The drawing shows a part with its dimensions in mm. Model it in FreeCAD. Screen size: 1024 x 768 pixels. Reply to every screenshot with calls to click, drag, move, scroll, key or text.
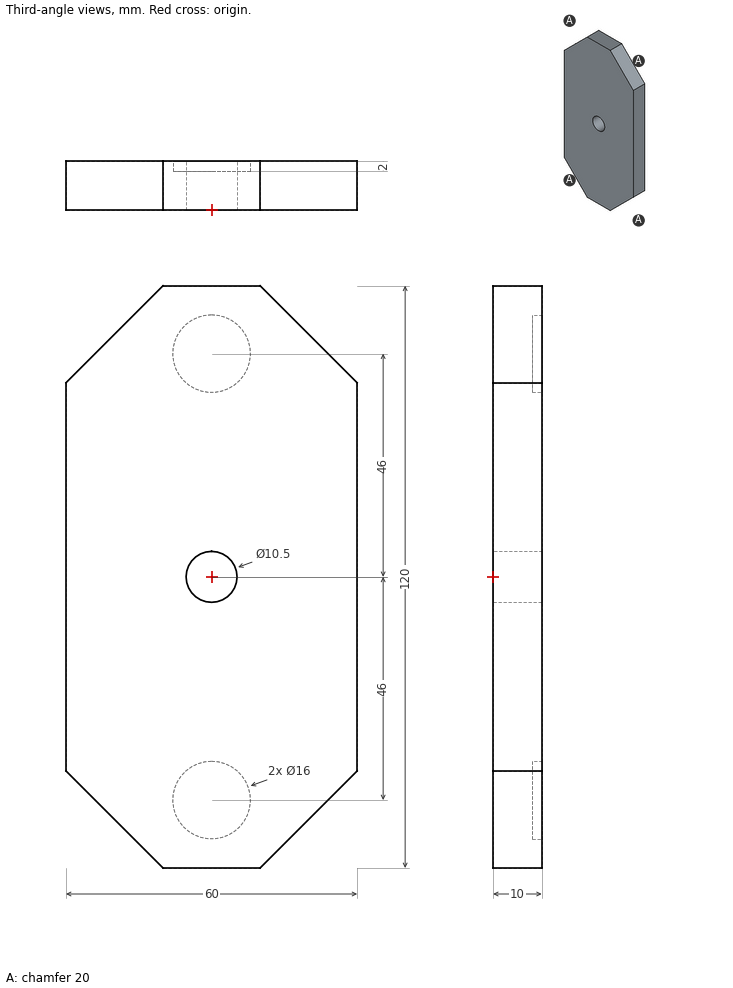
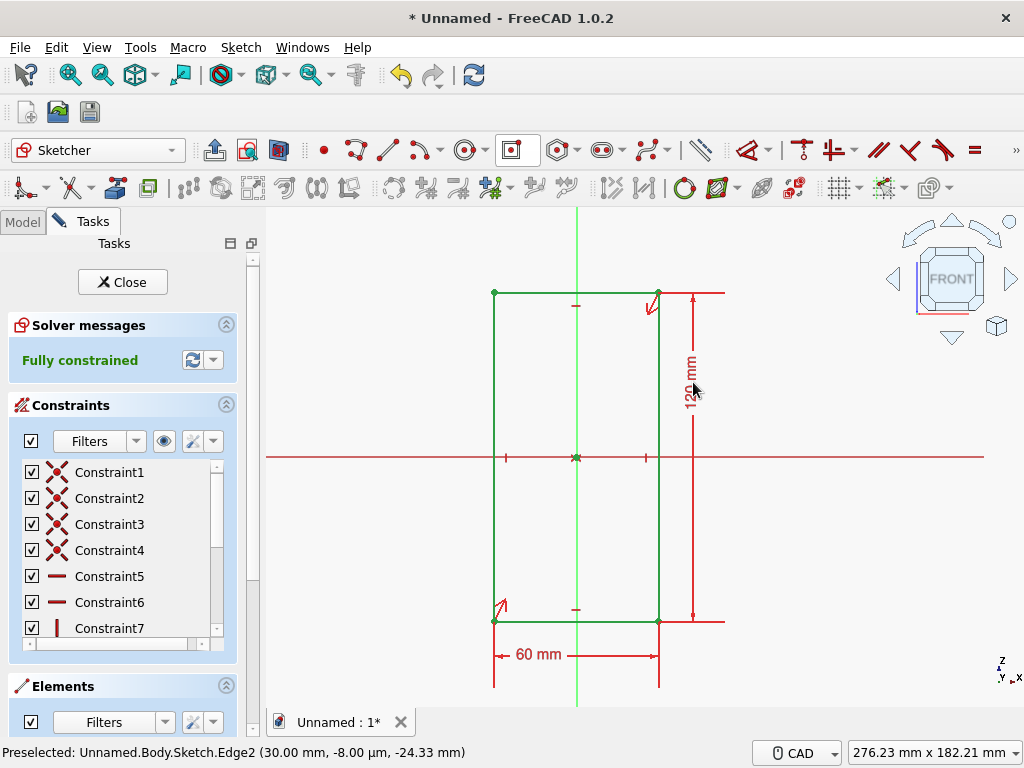
click(123, 282)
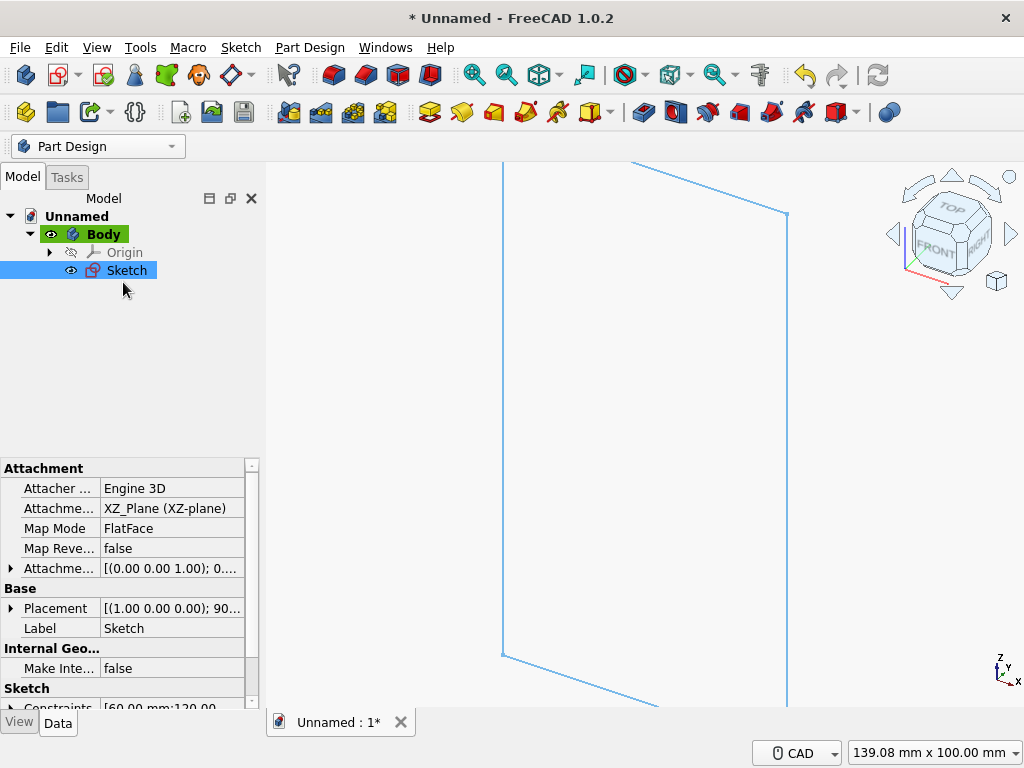
click(430, 112)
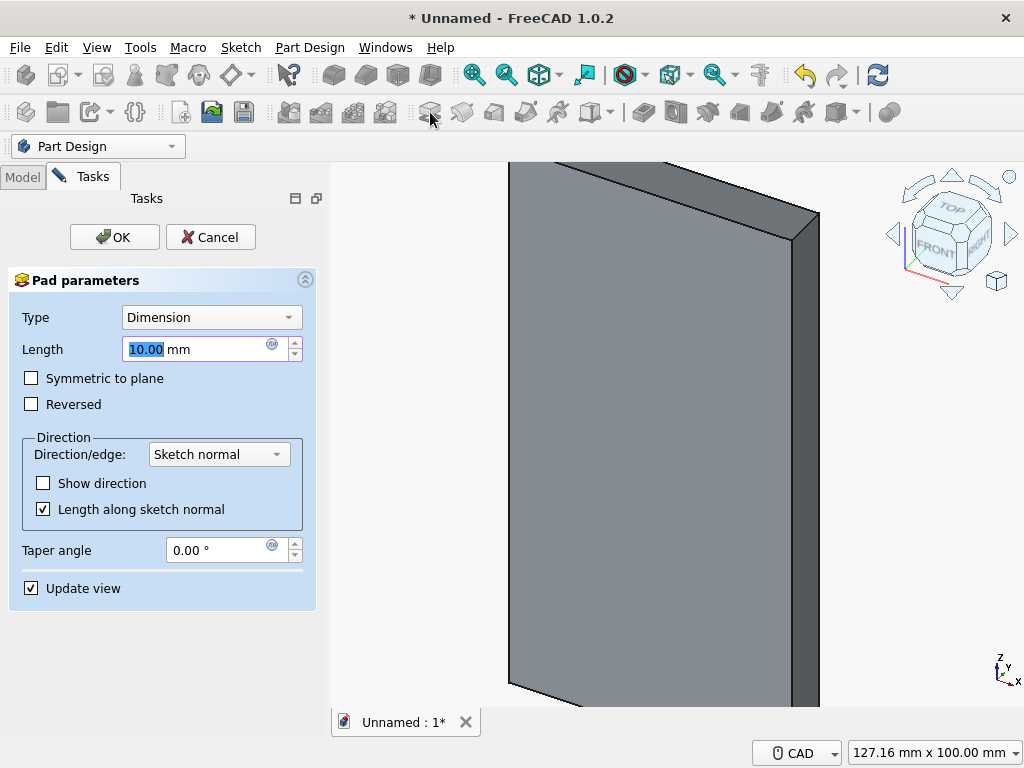
text(10)
key(Tab)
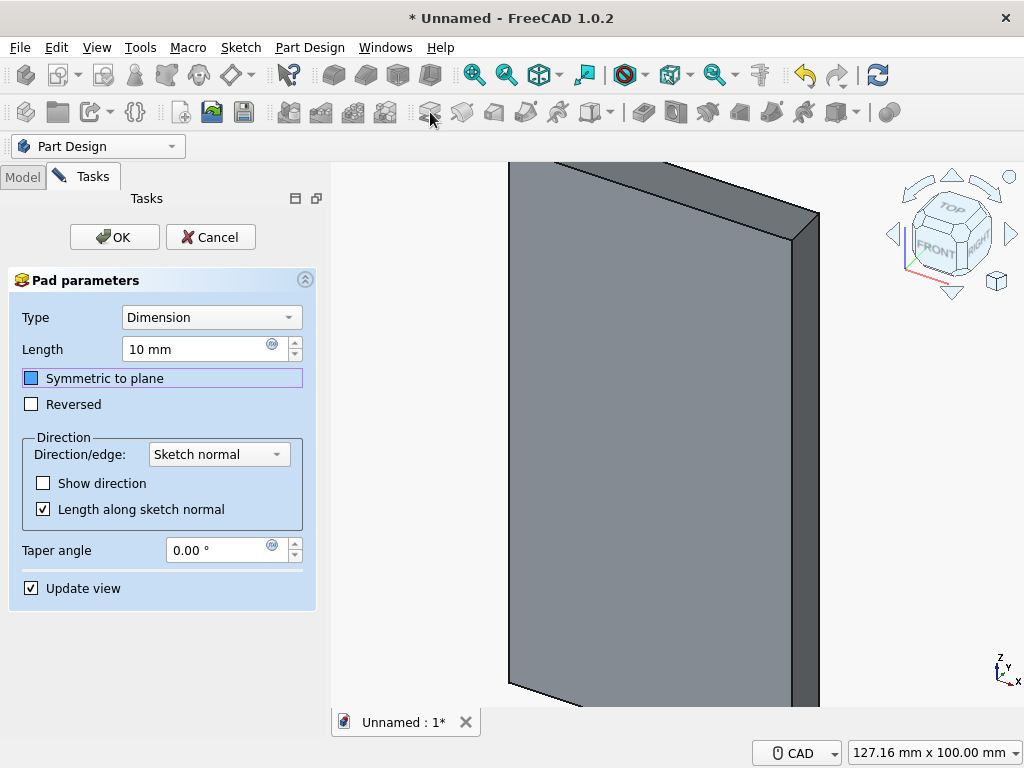
click(30, 404)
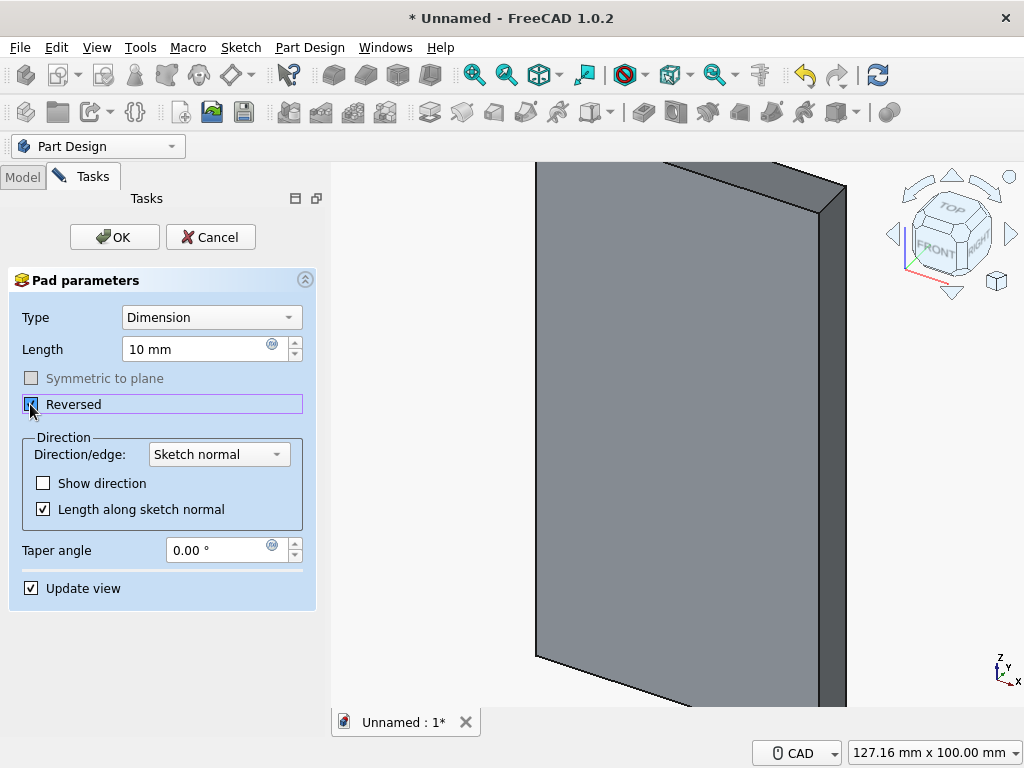
click(115, 237)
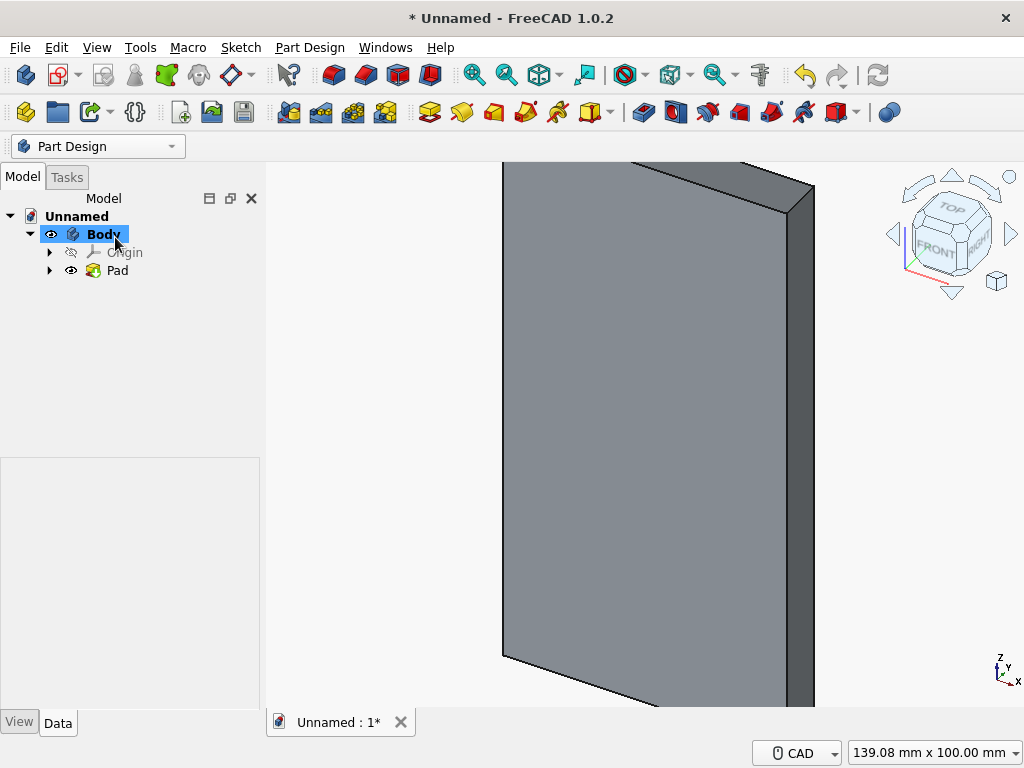
click(476, 76)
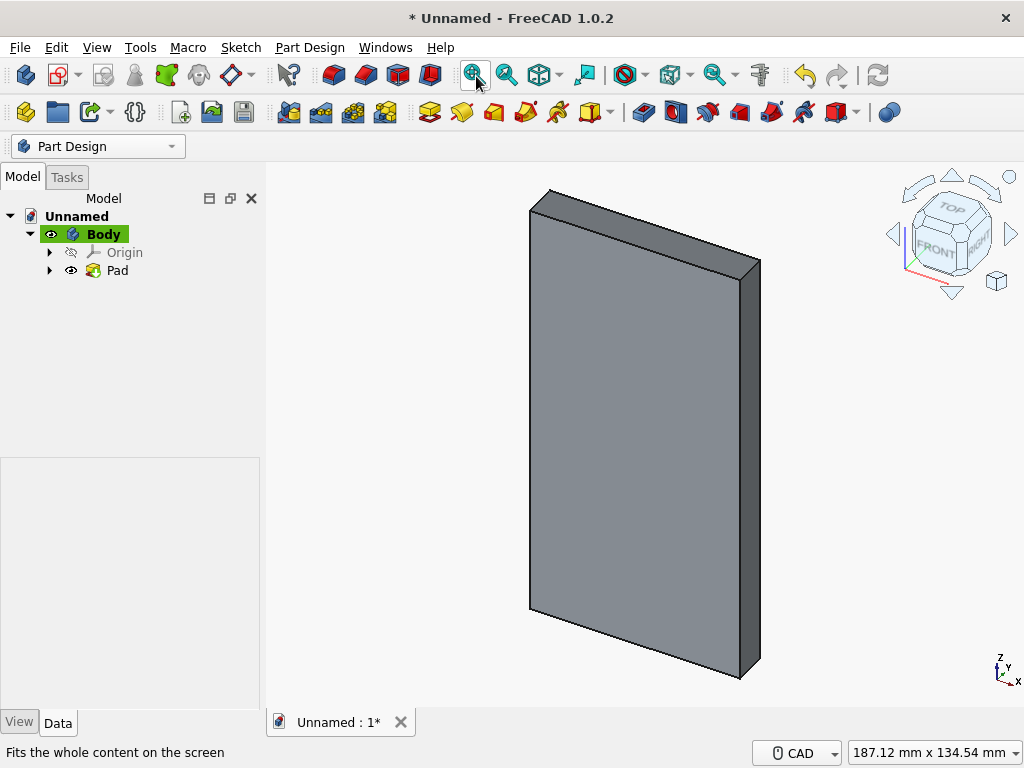
key(4)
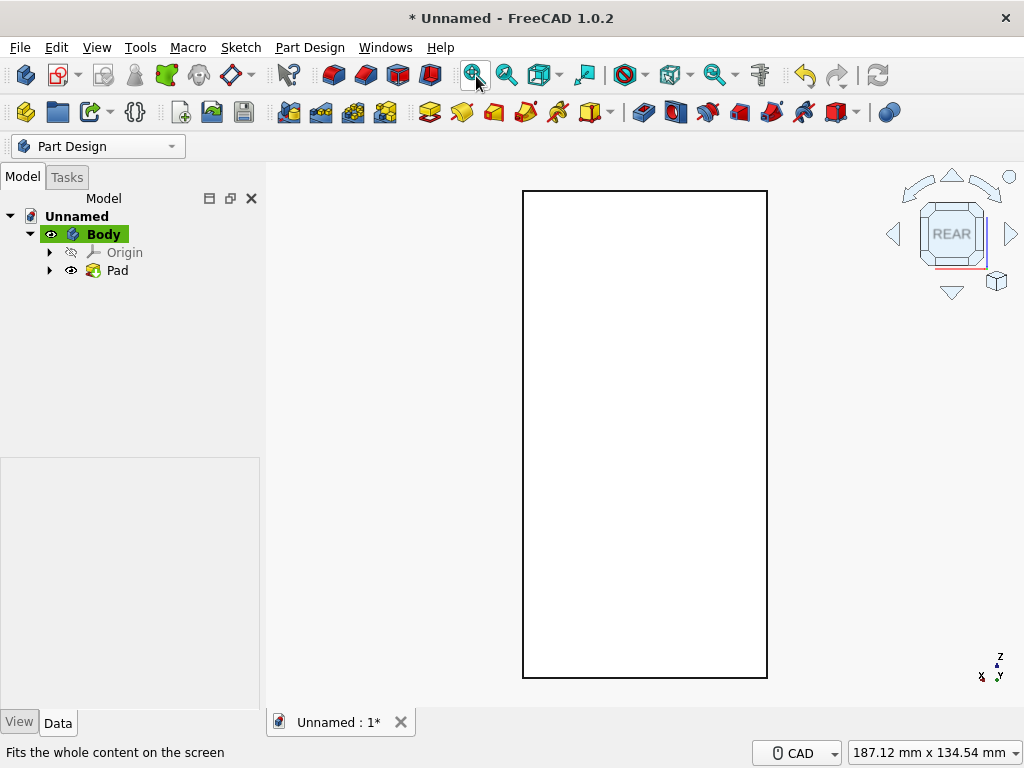
click(645, 364)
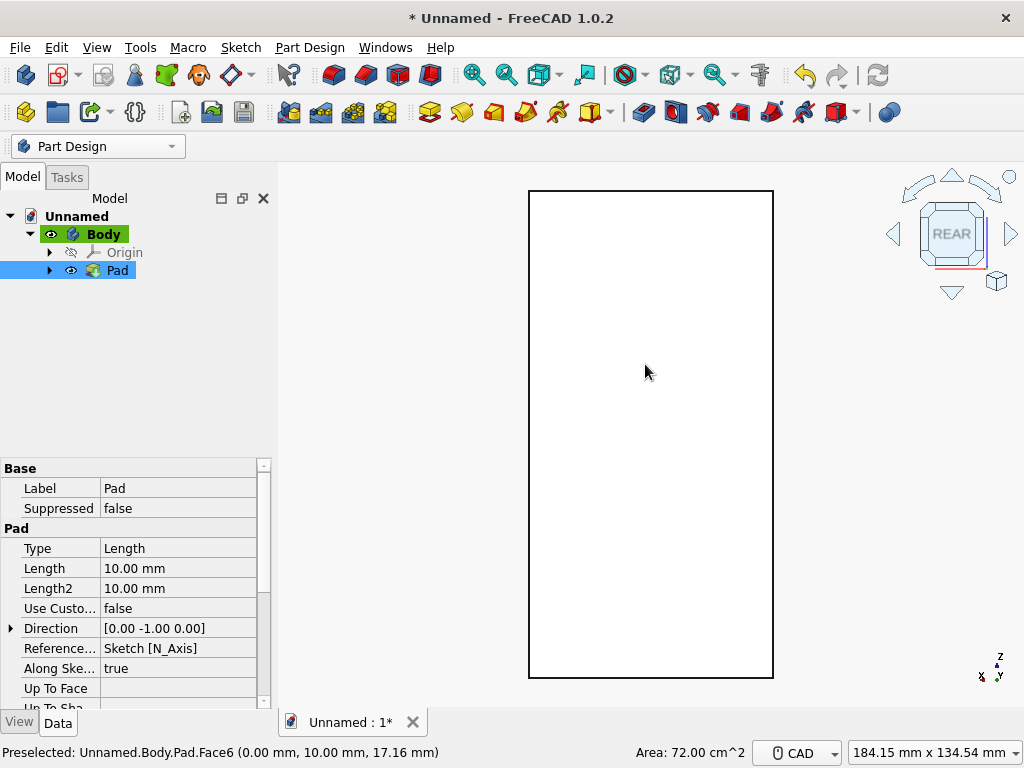
click(58, 76)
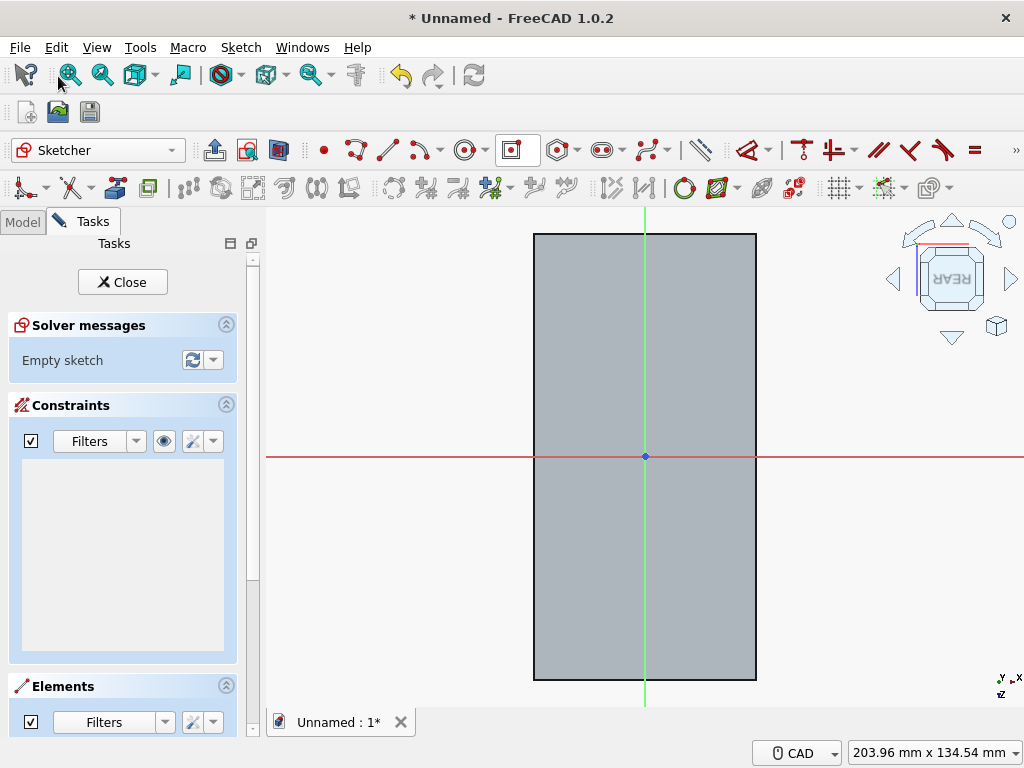
scroll(294, 457, down, 1)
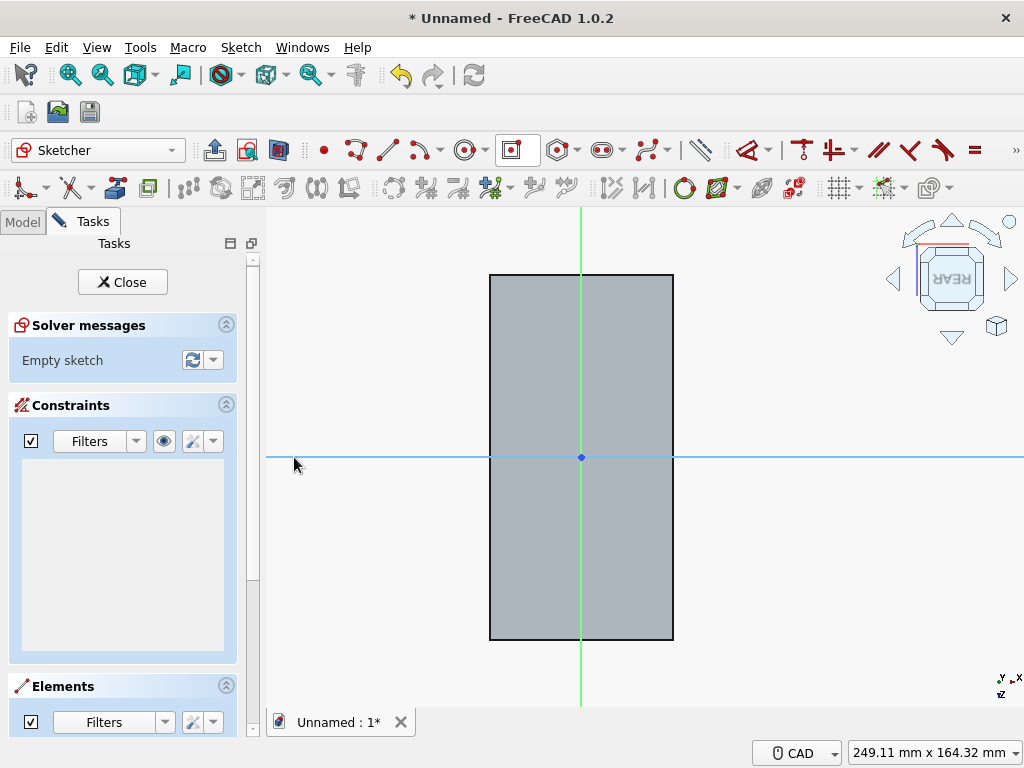
click(466, 150)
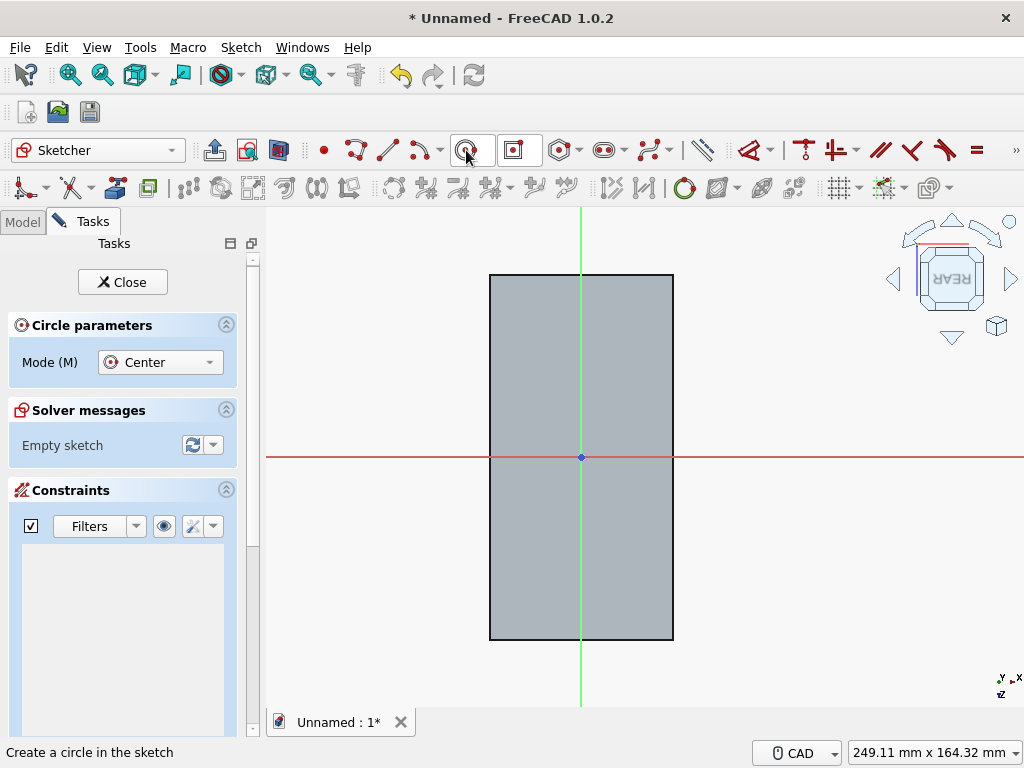
click(581, 317)
click(599, 300)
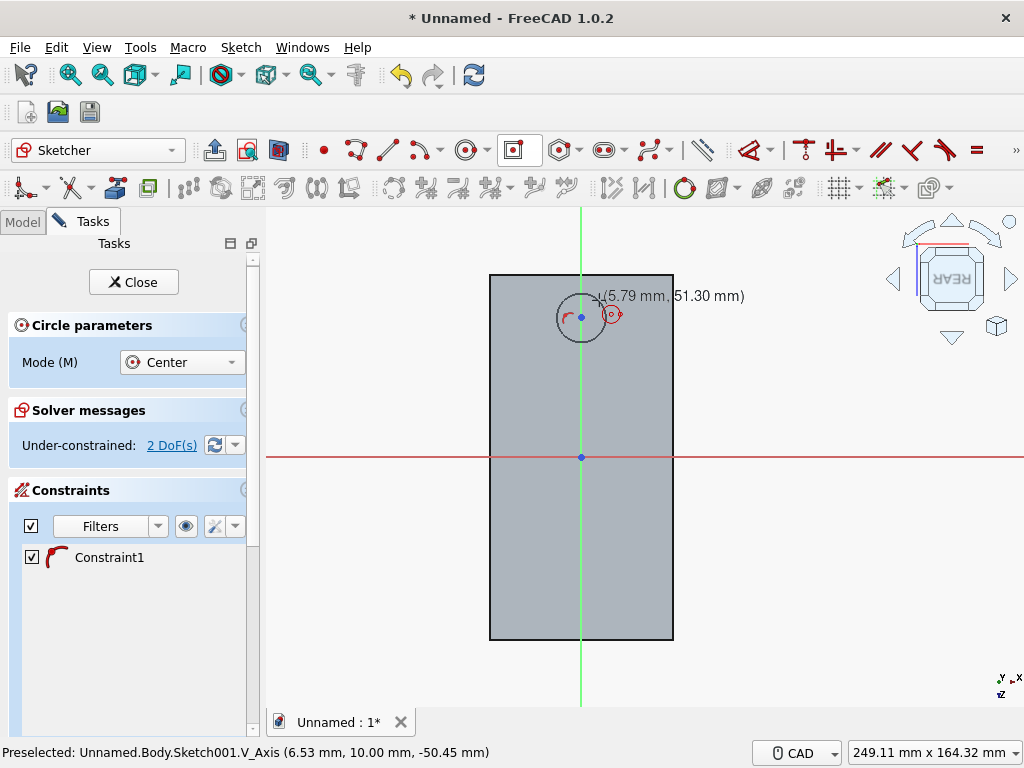
click(581, 597)
click(599, 580)
key(Escape)